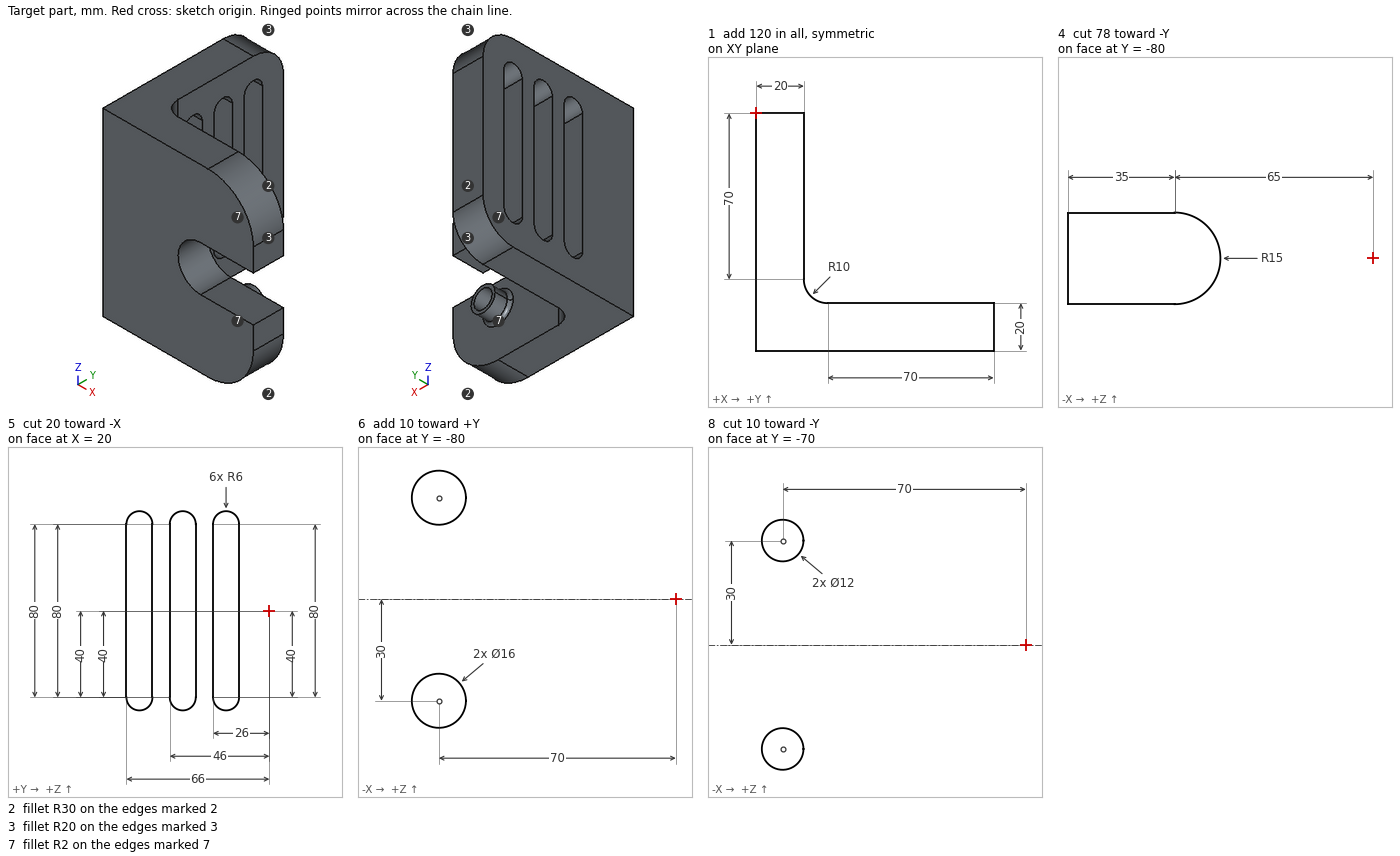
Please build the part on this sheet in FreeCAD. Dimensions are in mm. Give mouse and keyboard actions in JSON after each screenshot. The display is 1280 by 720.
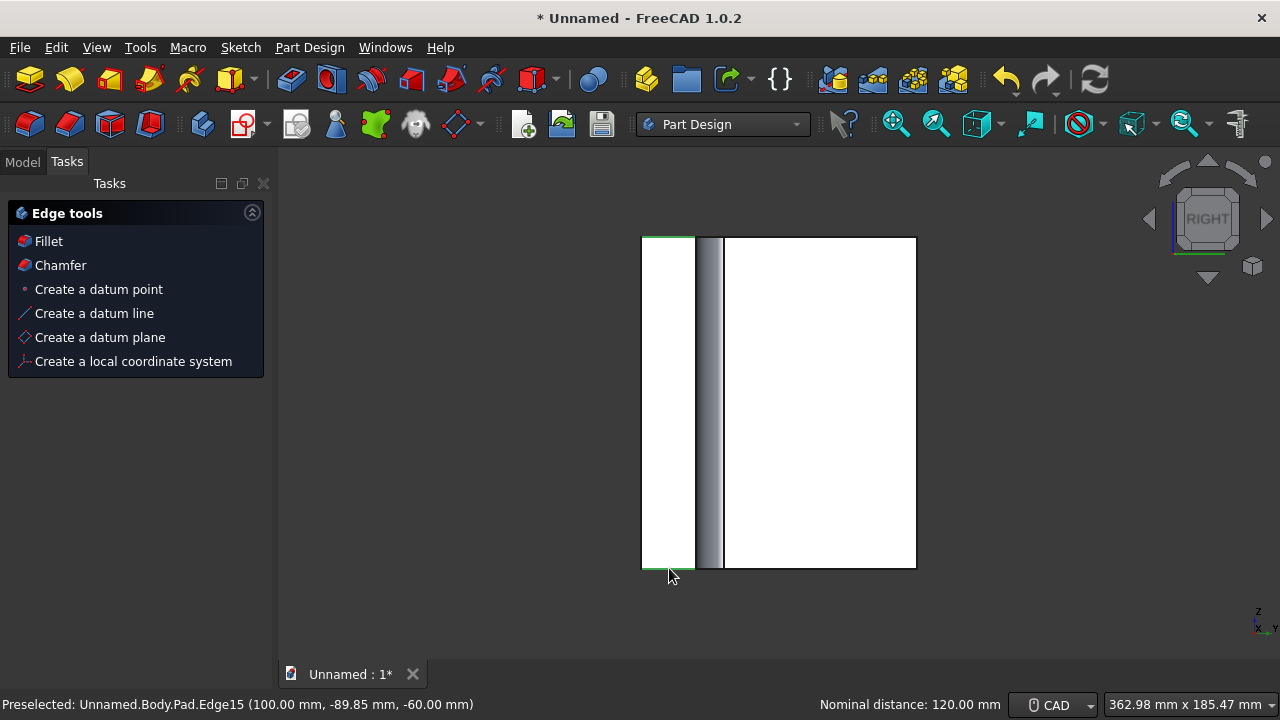
{"action": "left_click", "coordinate": [30, 124]}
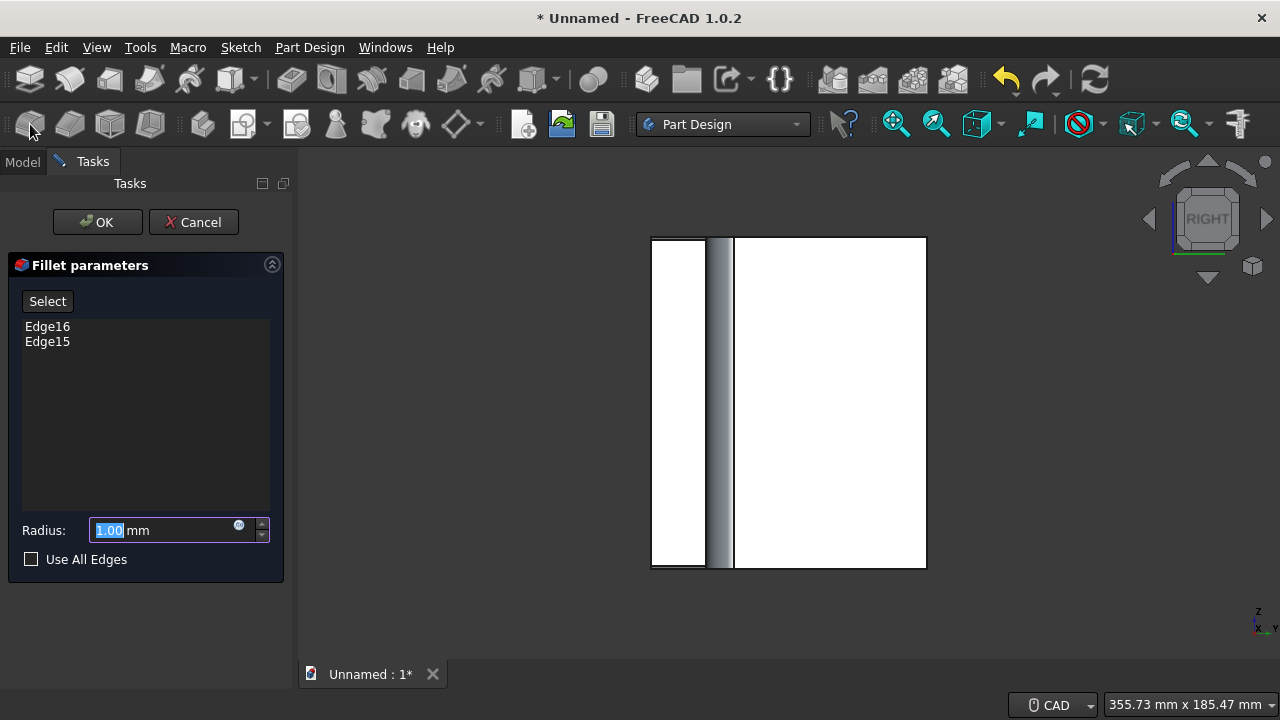
{"action": "type", "text": "30"}
{"action": "key", "text": "Tab"}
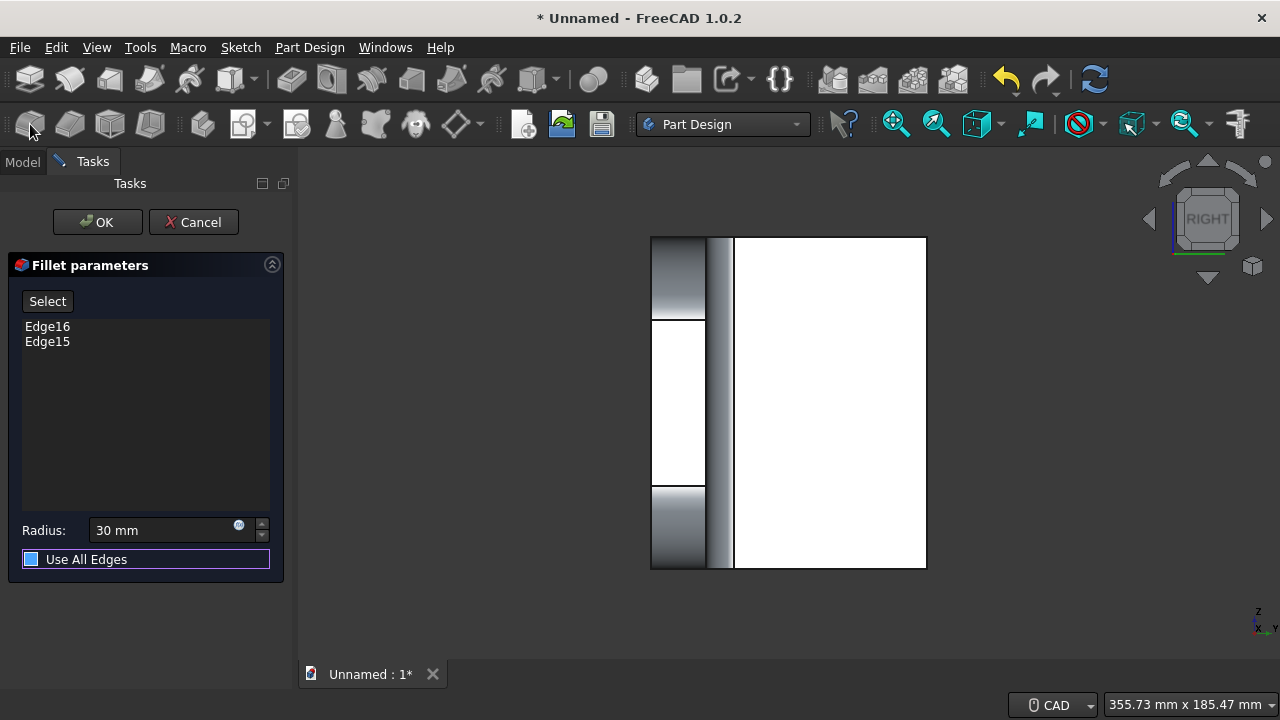
{"action": "left_click", "coordinate": [98, 222]}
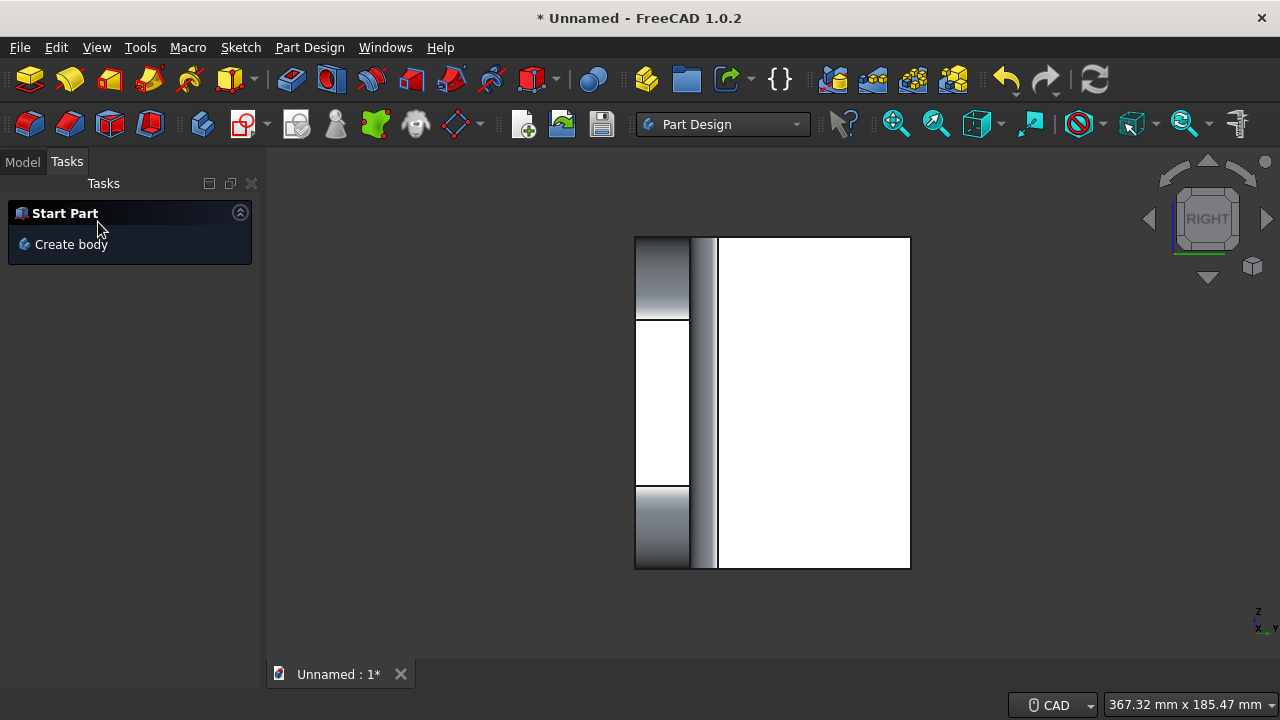
{"action": "key", "text": "0"}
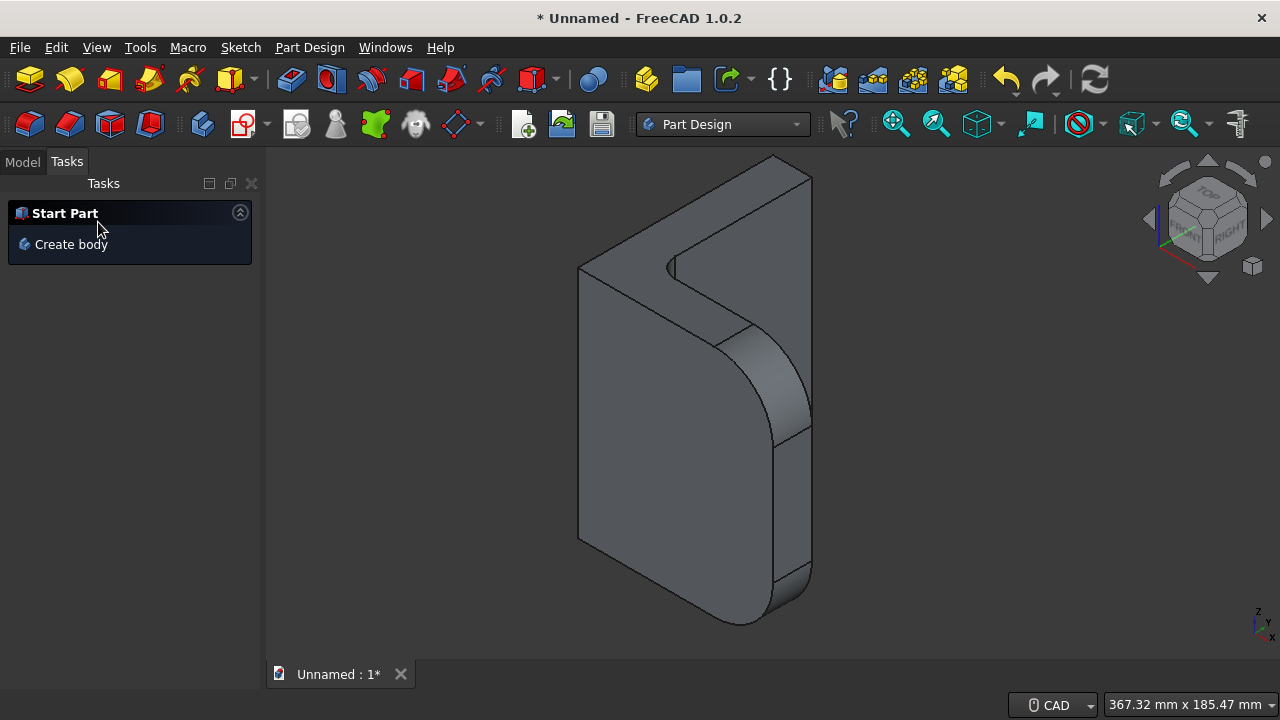
{"action": "key", "text": "2"}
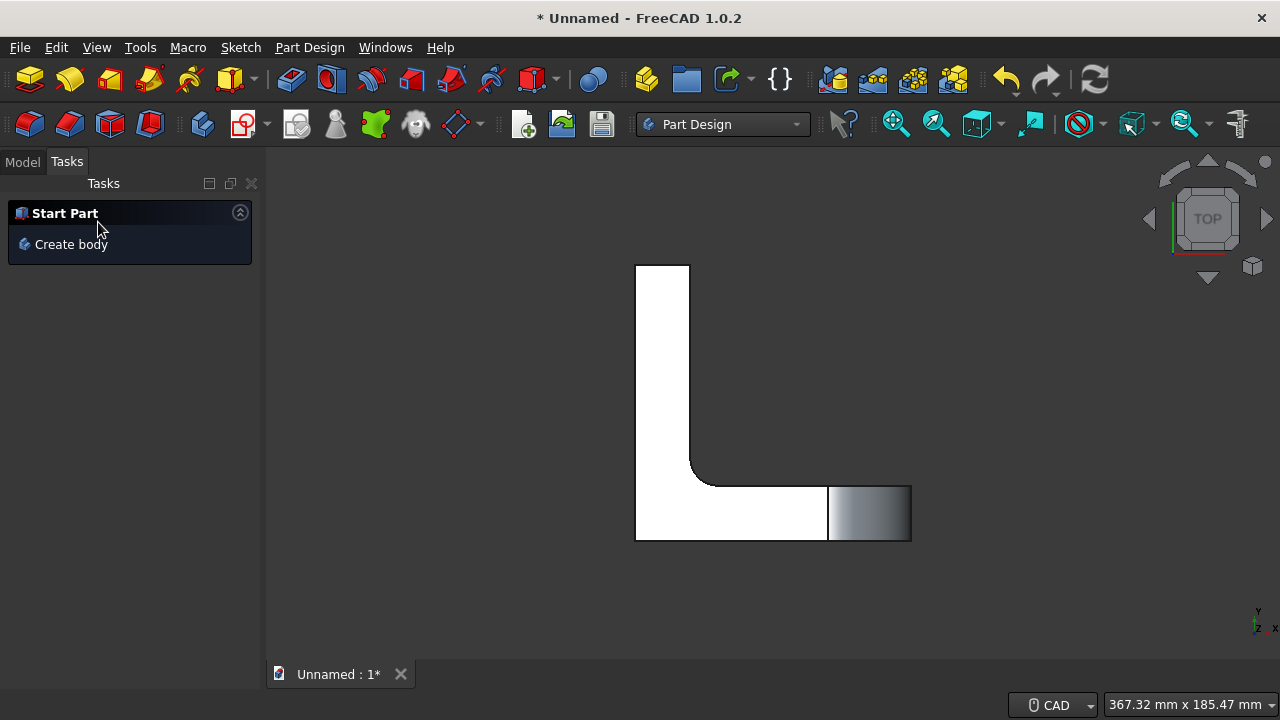
{"action": "left_click", "coordinate": [663, 264]}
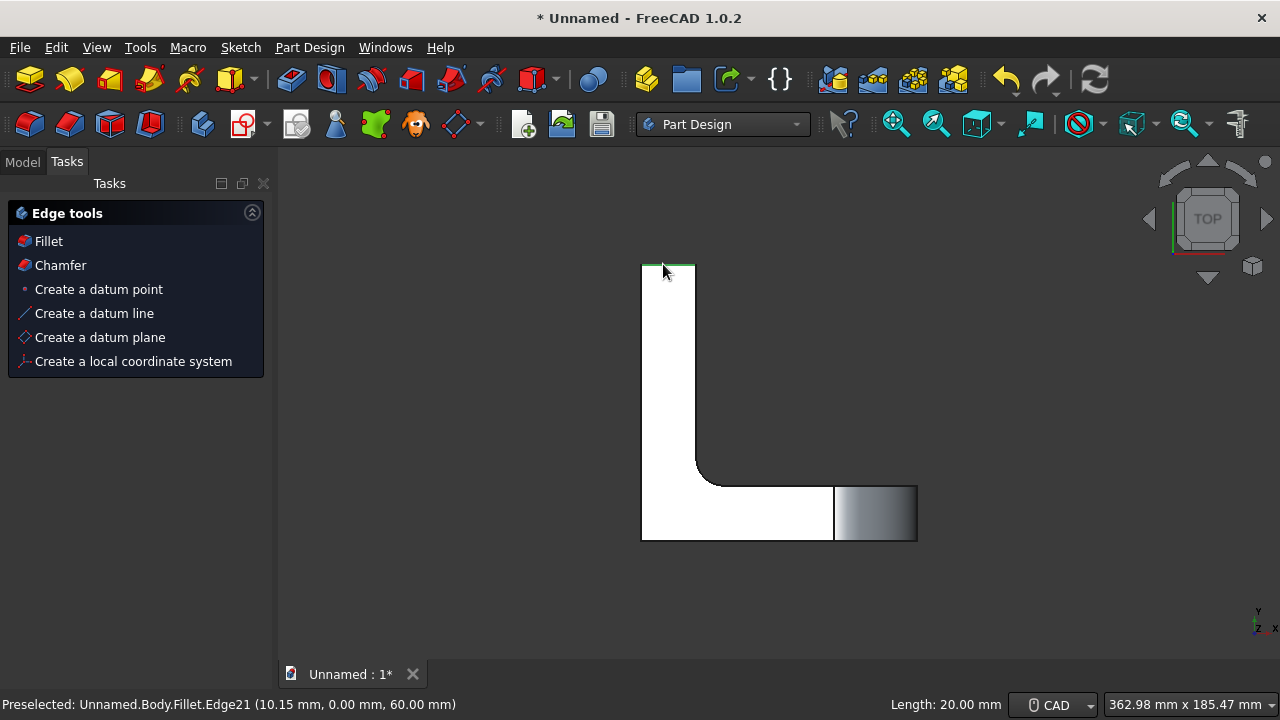
{"action": "key", "text": "1"}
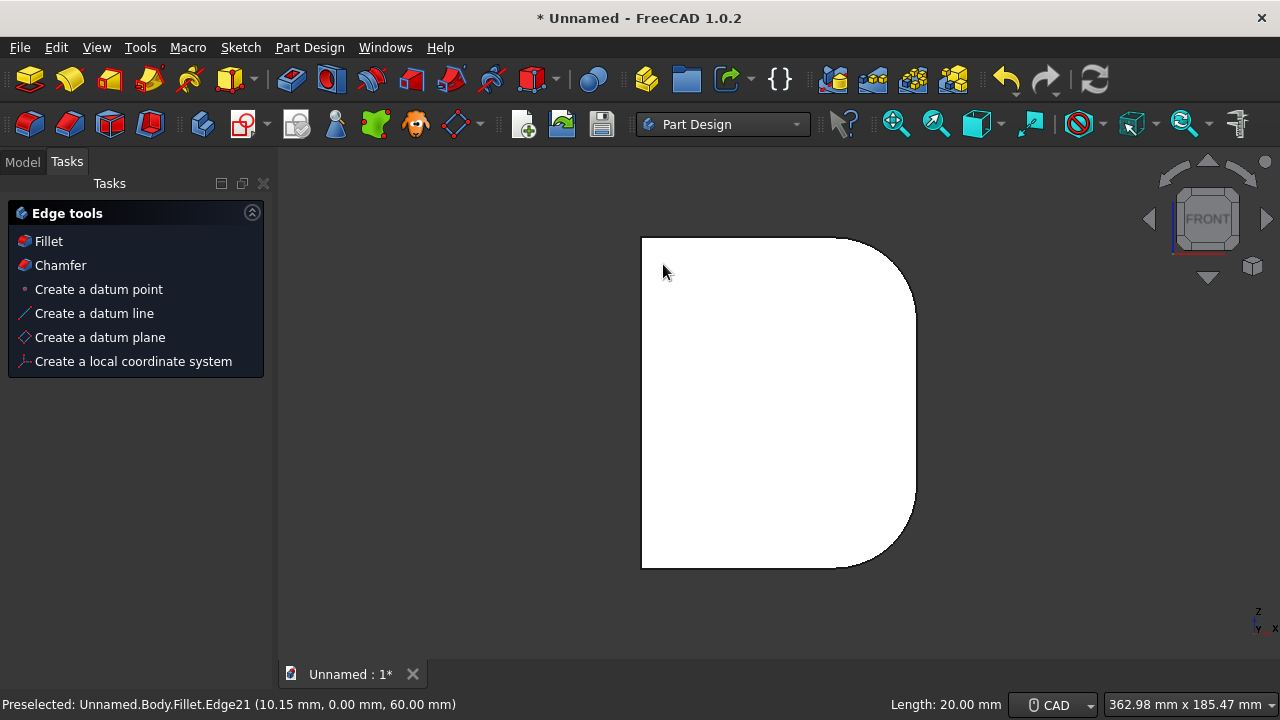
{"action": "key", "text": "3"}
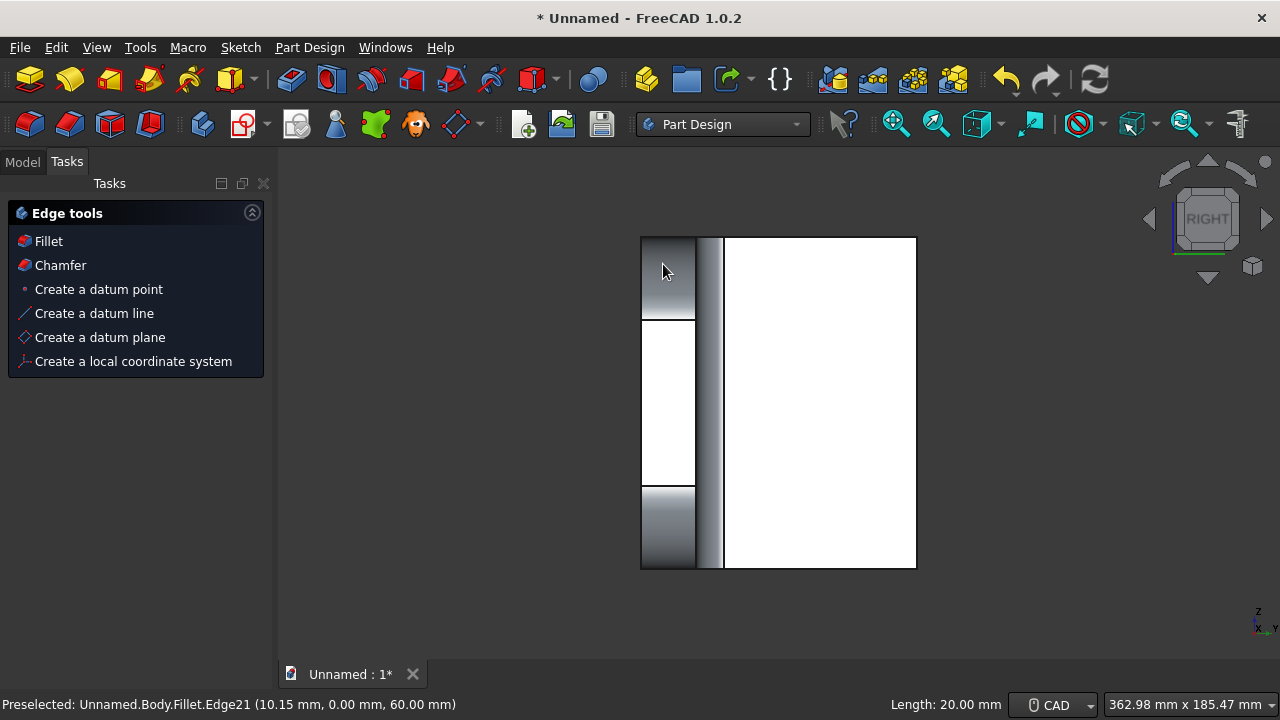
{"action": "key", "text": "5"}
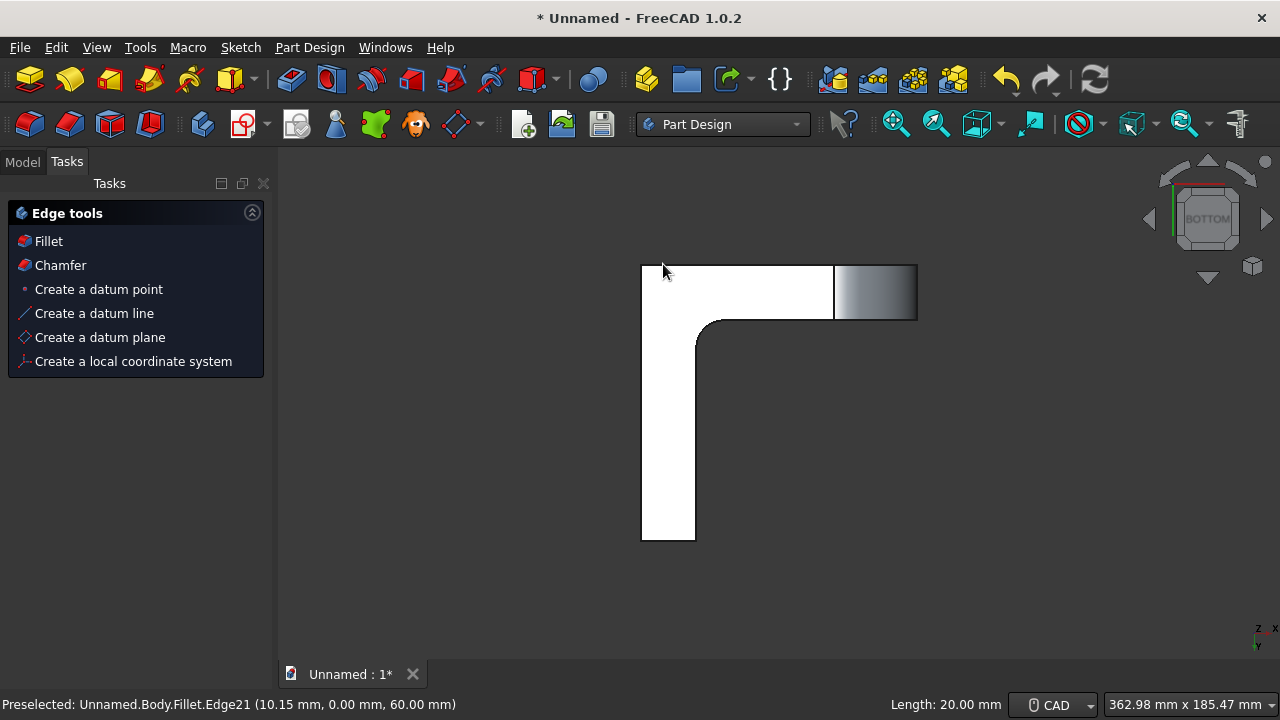
{"action": "left_click", "coordinate": [669, 540], "text": "ctrl"}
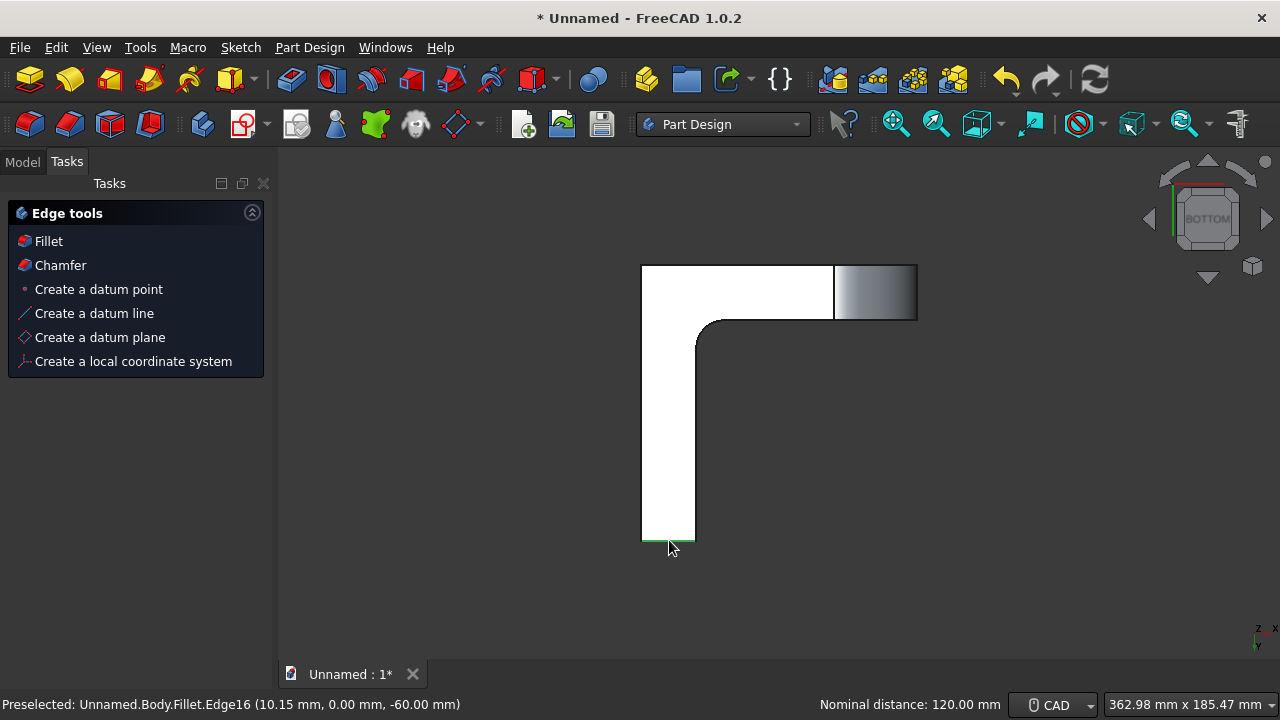
{"action": "left_click", "coordinate": [30, 124]}